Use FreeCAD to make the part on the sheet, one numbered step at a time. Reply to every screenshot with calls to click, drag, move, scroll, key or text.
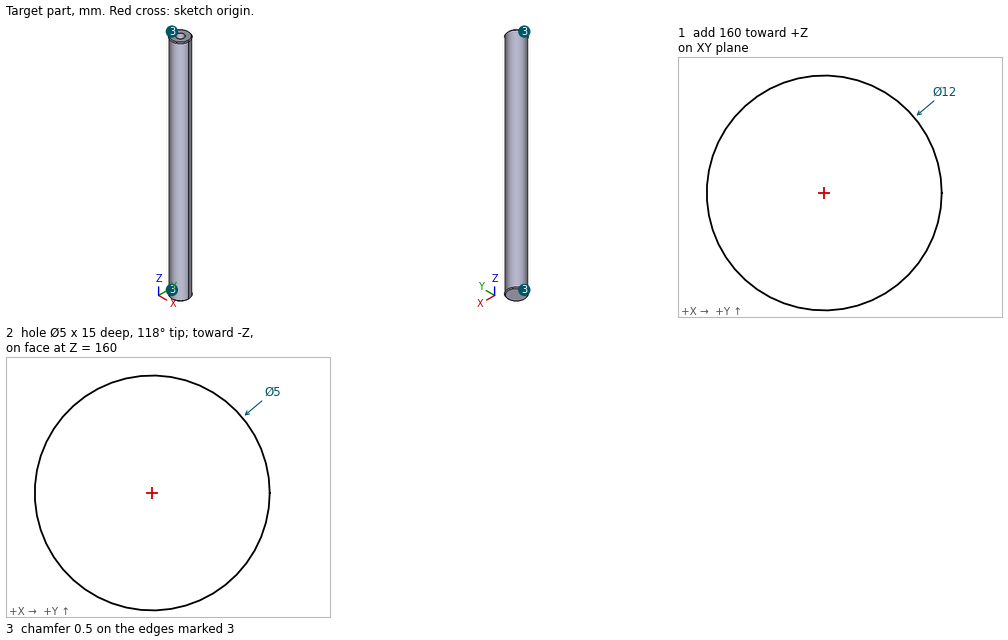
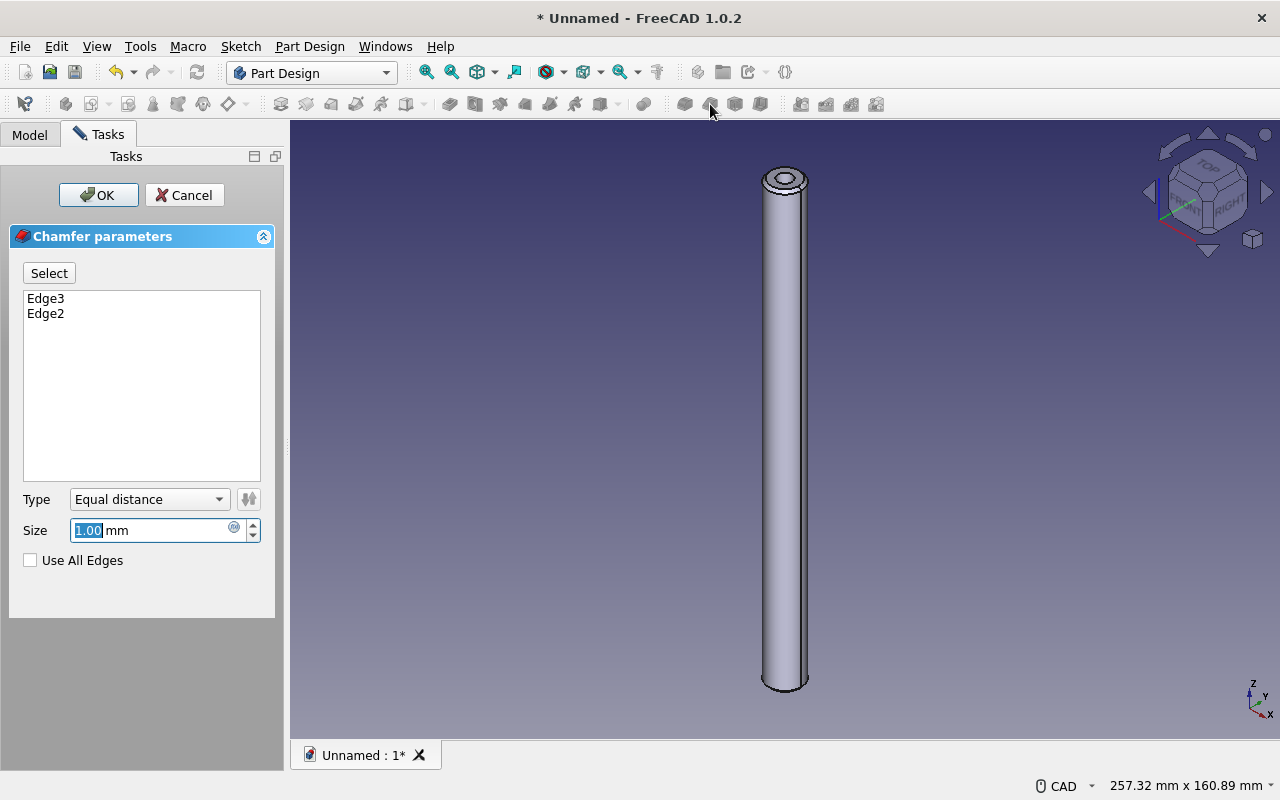
text(0.5)
key(Tab)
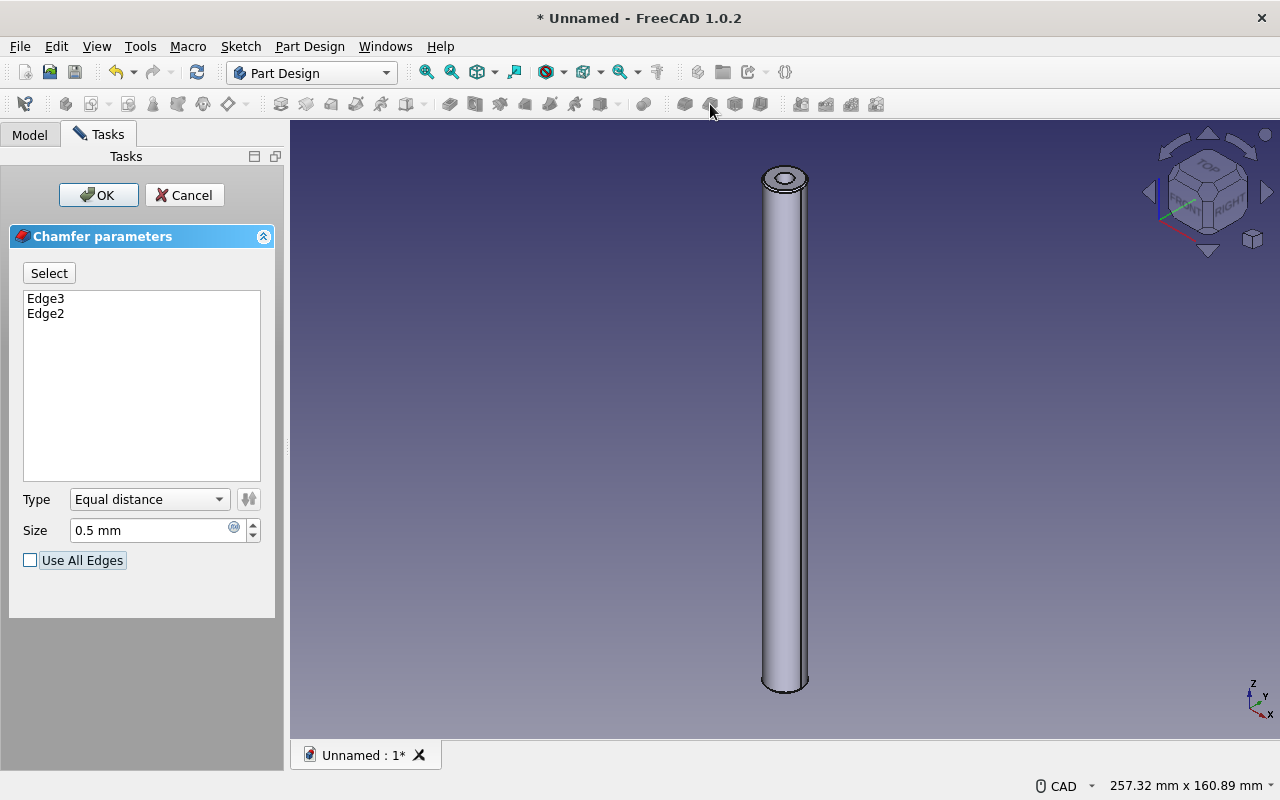
click(99, 195)